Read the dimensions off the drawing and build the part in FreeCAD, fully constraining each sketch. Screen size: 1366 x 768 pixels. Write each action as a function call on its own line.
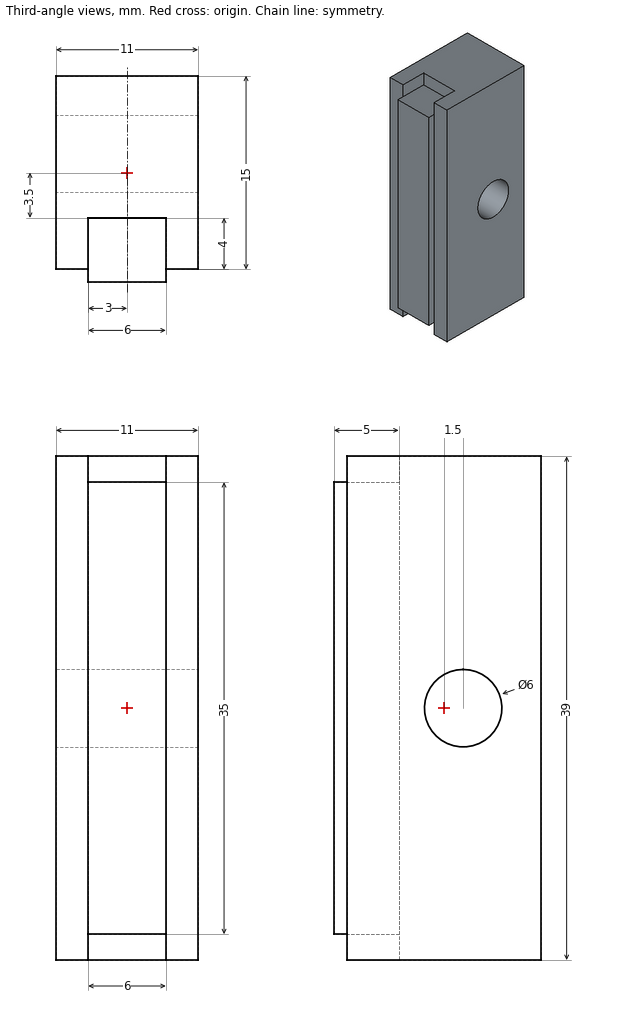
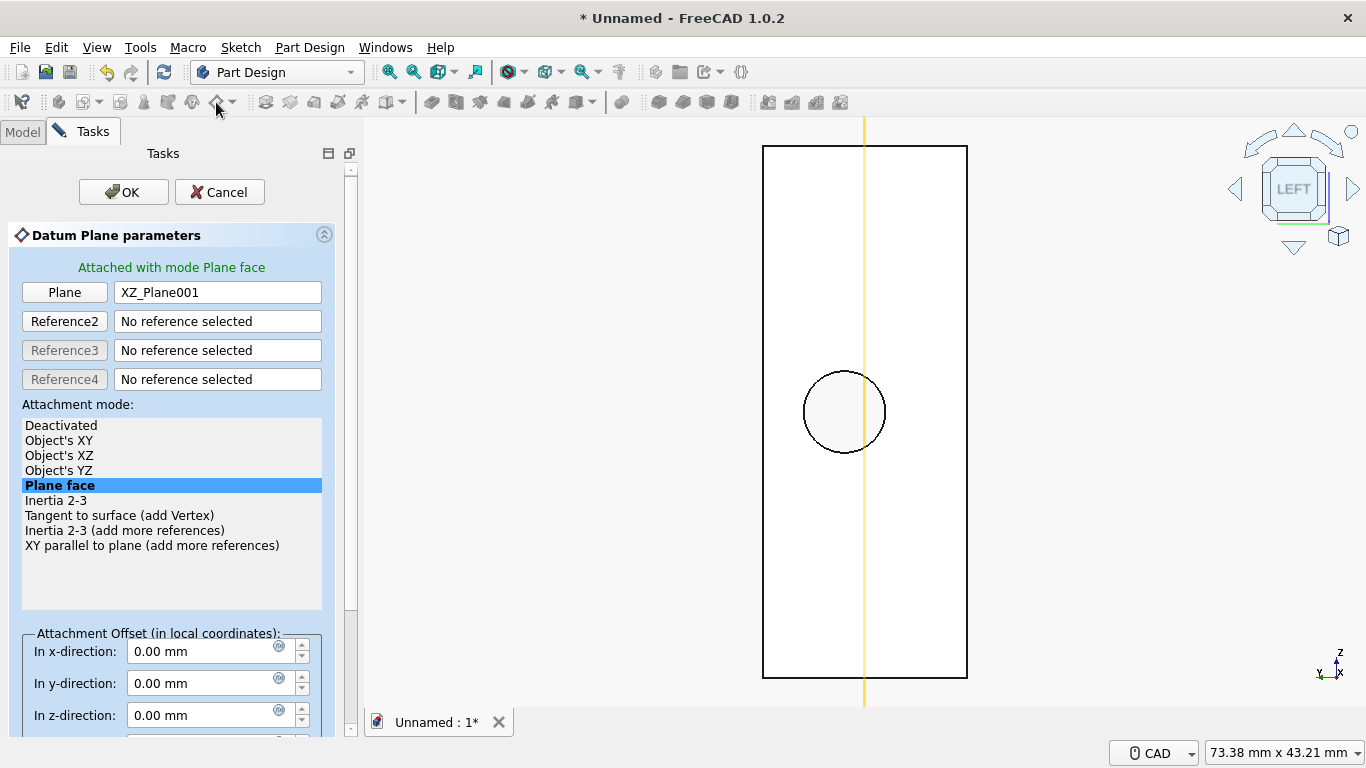
triple_click(210, 715)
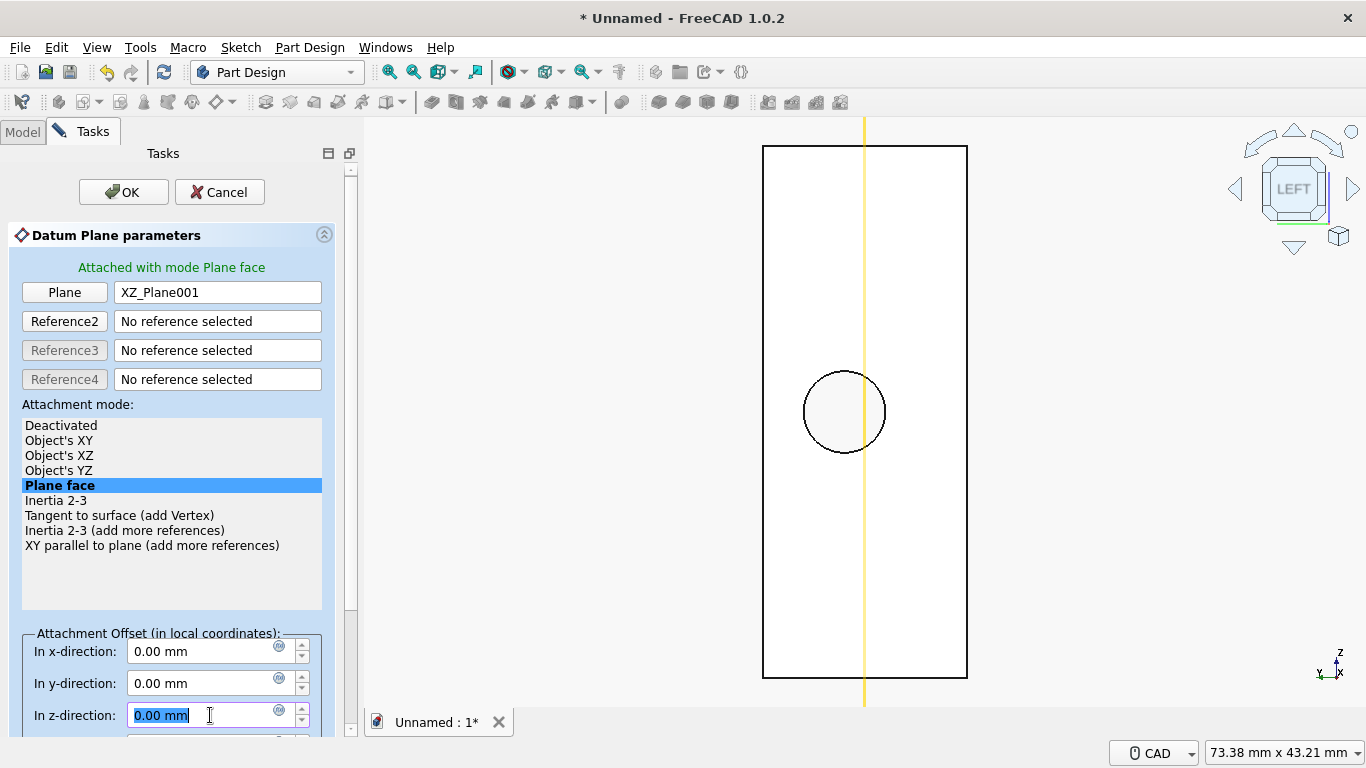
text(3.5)
key(Tab)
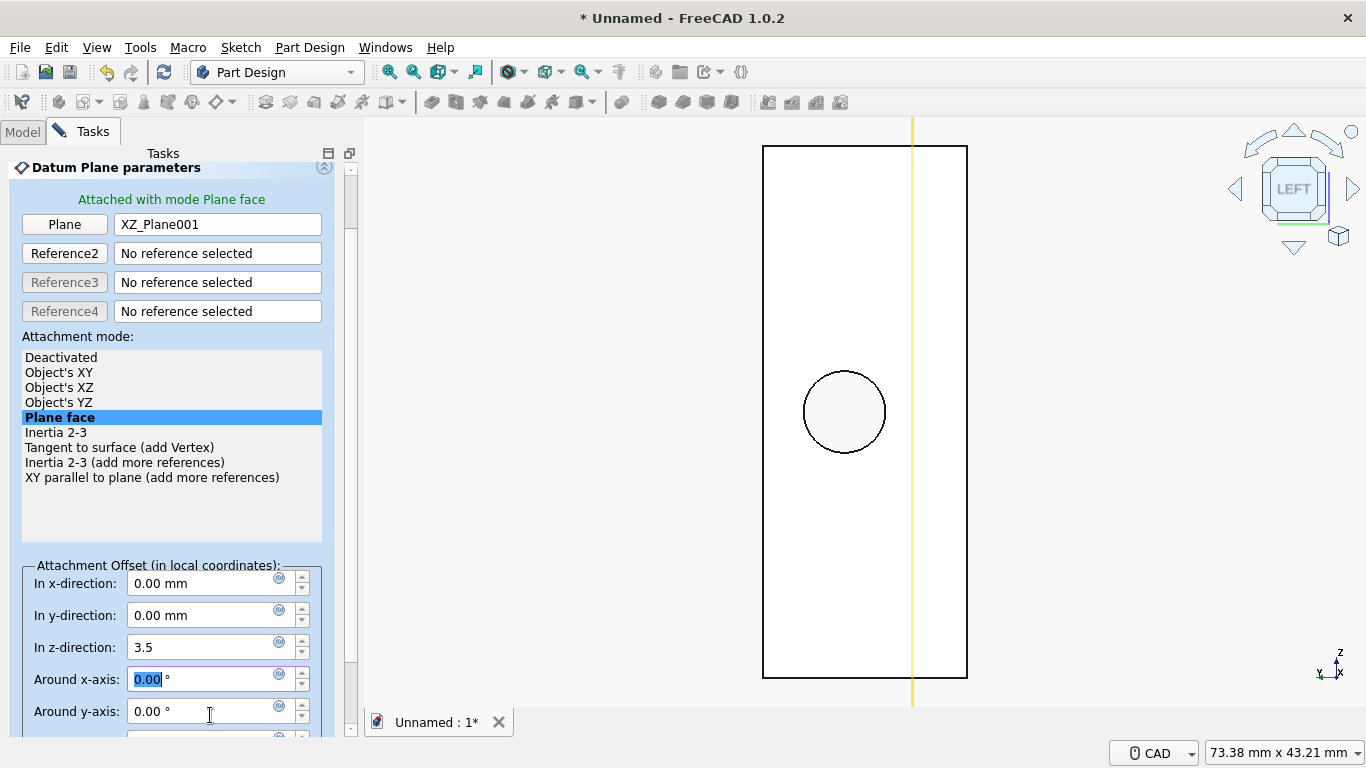
scroll(351, 450, up, 2)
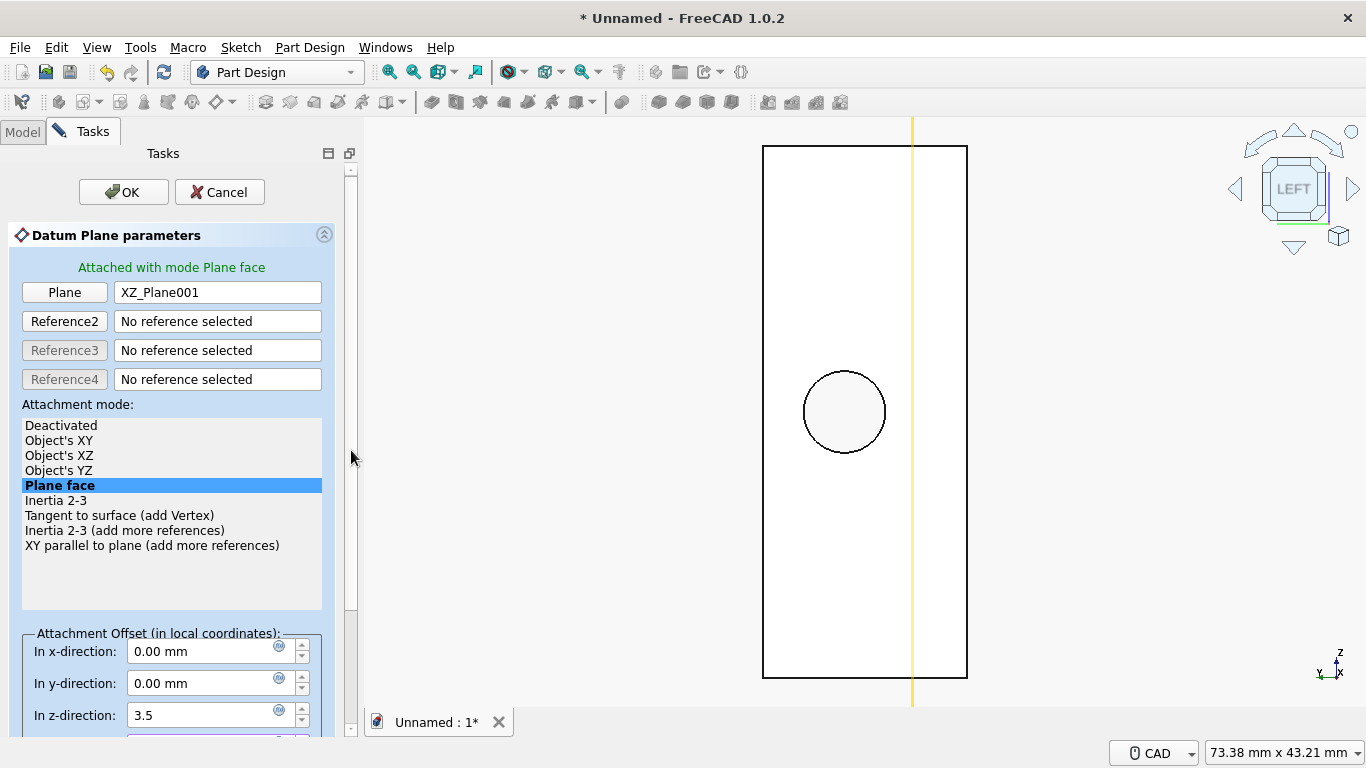
click(124, 192)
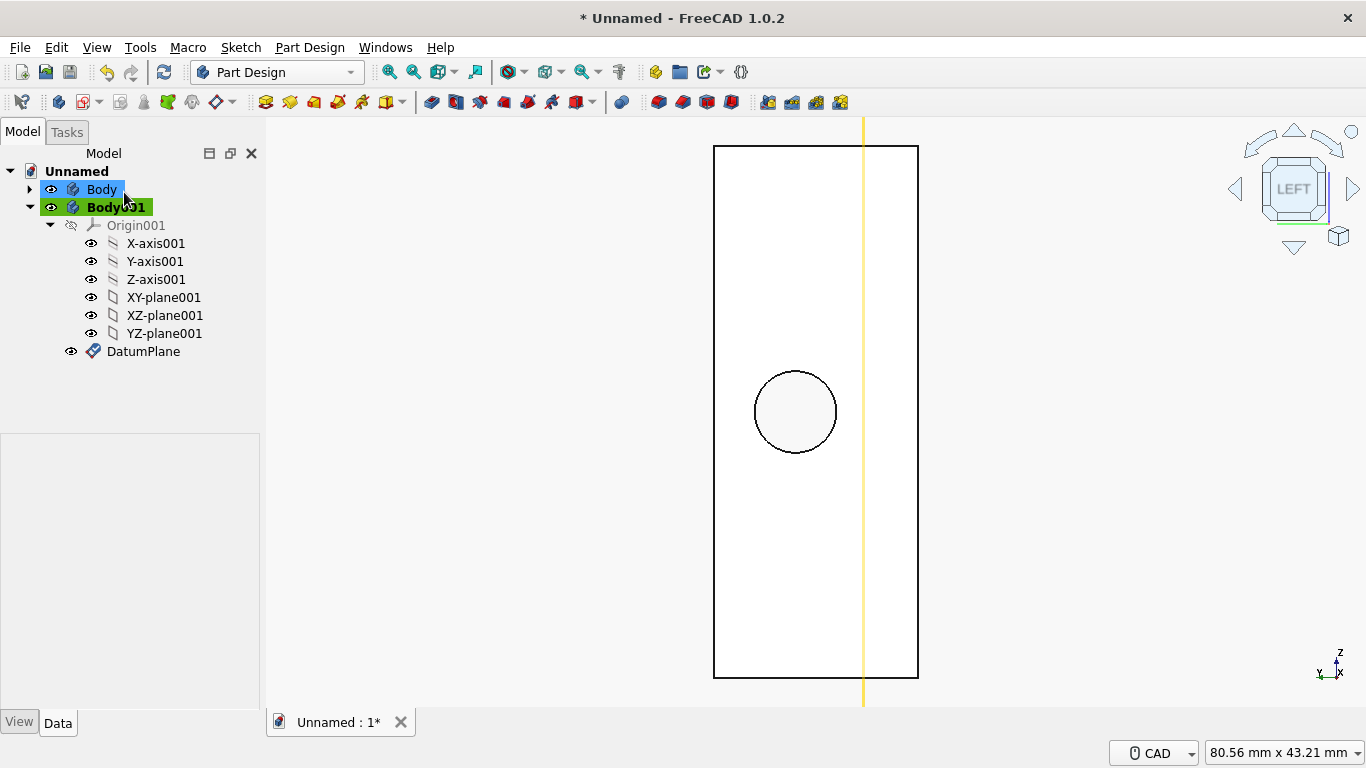
click(116, 351)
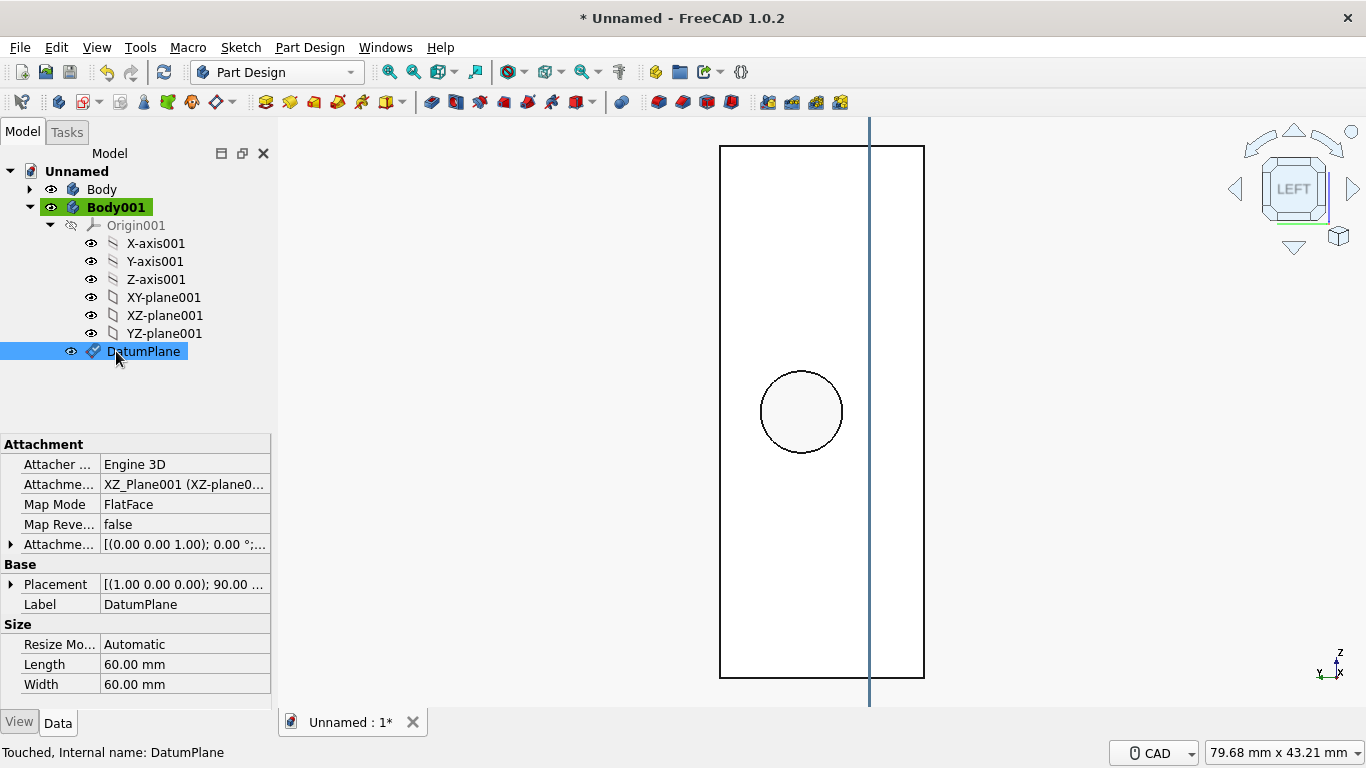
click(84, 102)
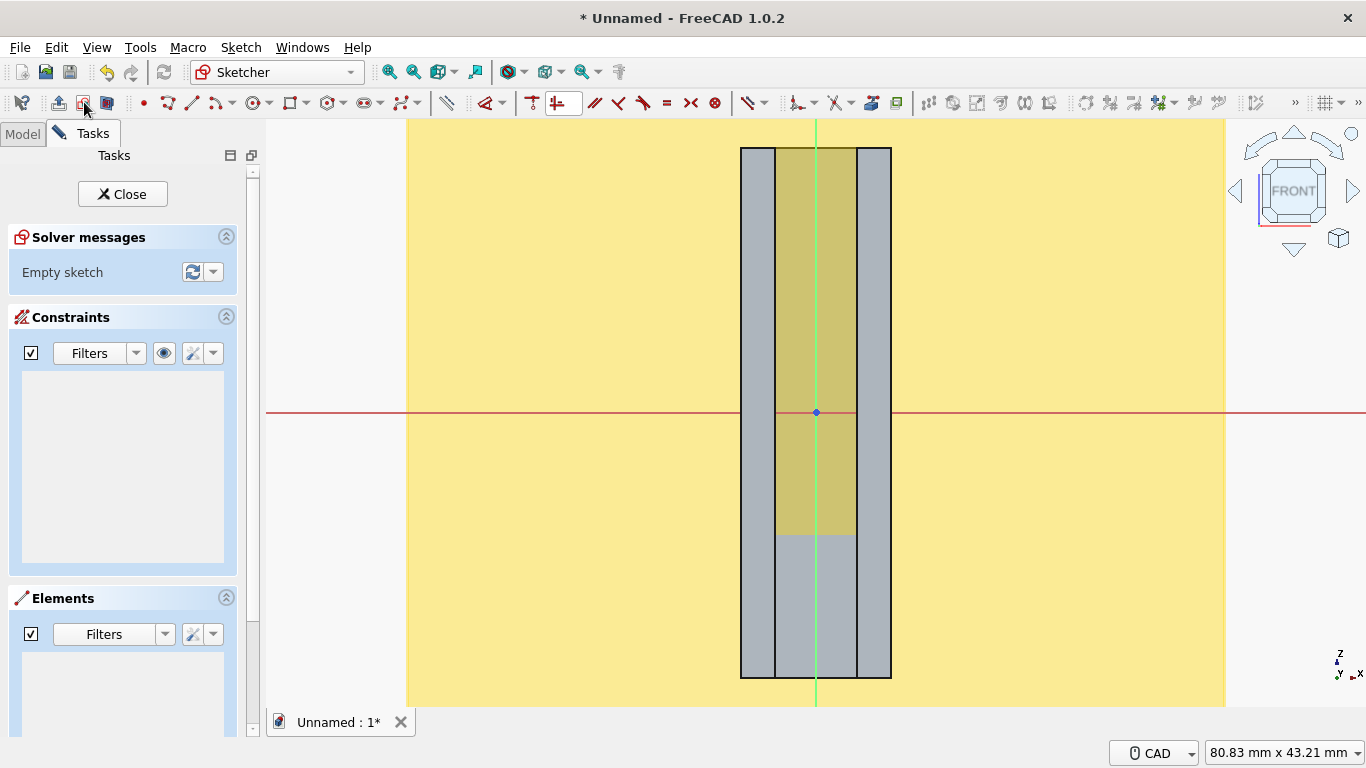
click(308, 104)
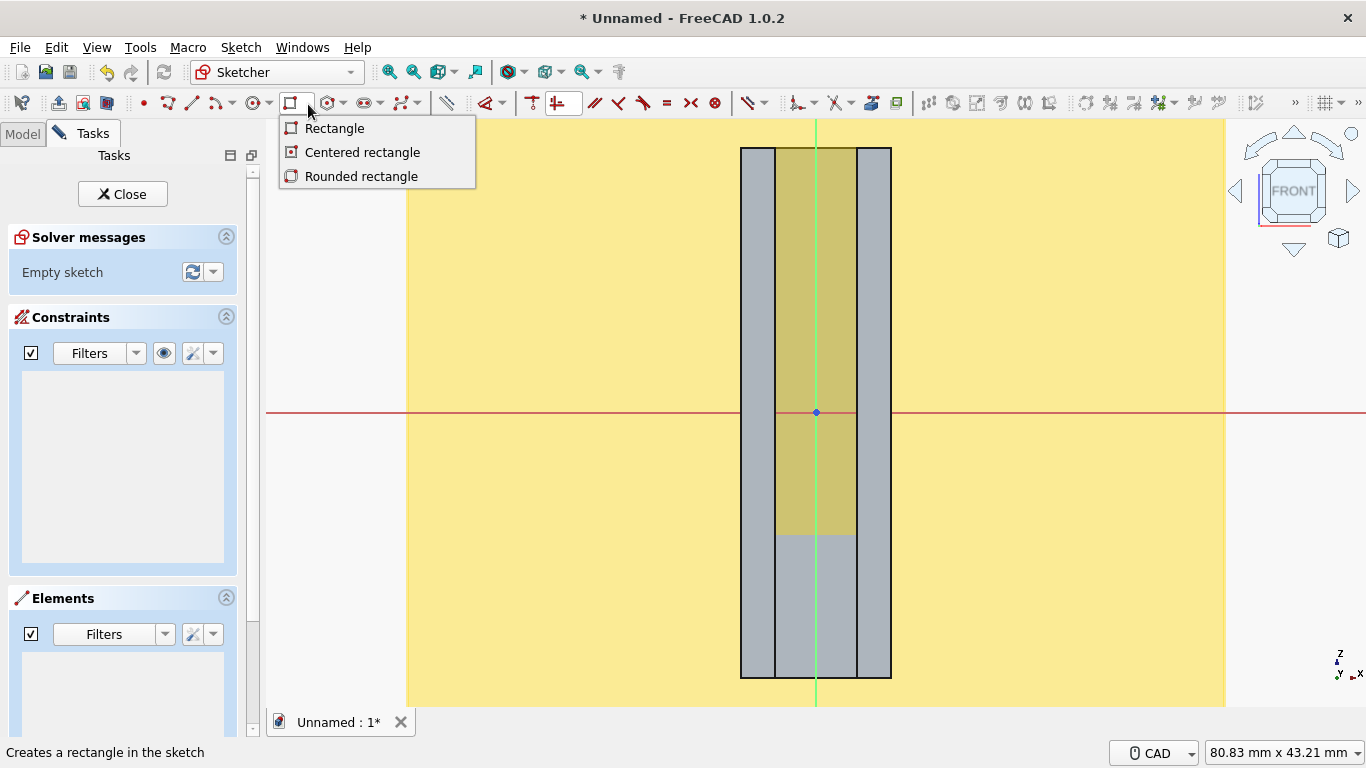
click(378, 152)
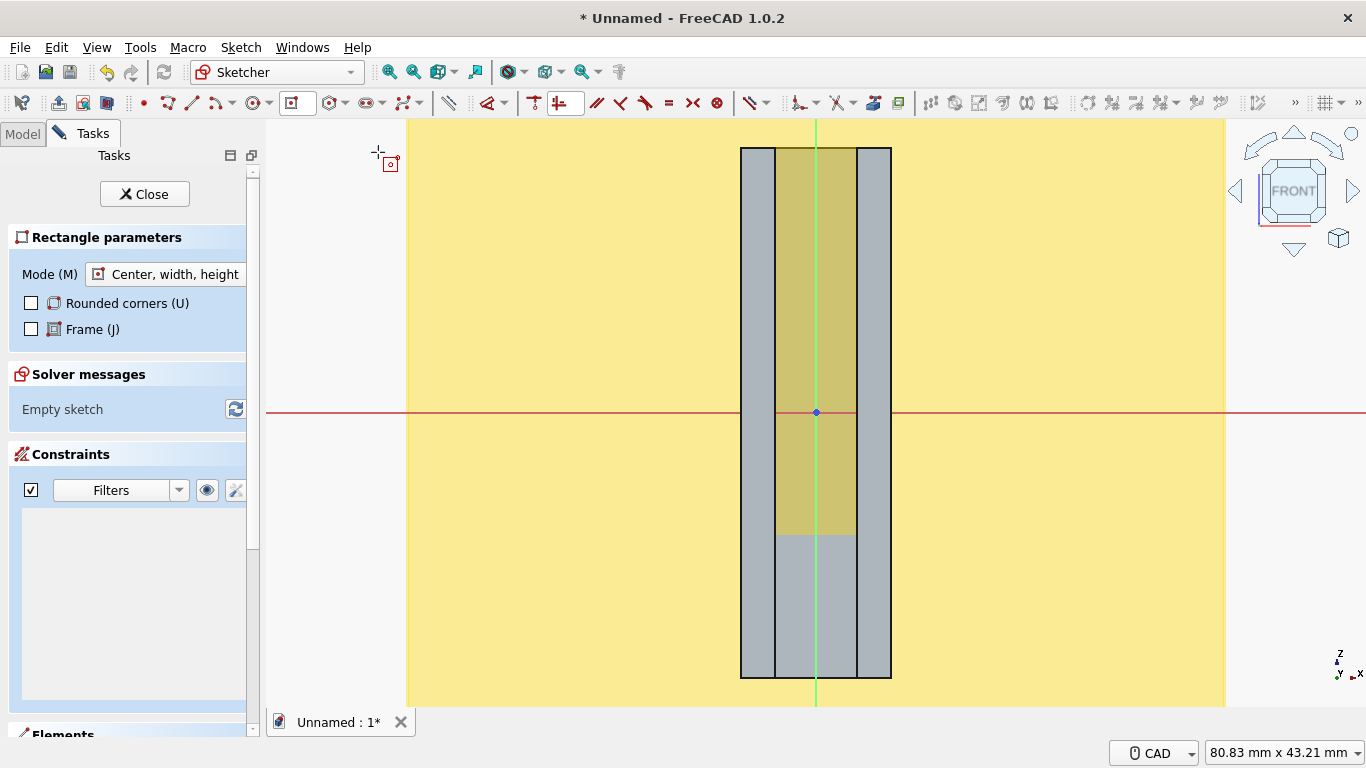
click(816, 413)
click(857, 175)
key(Escape)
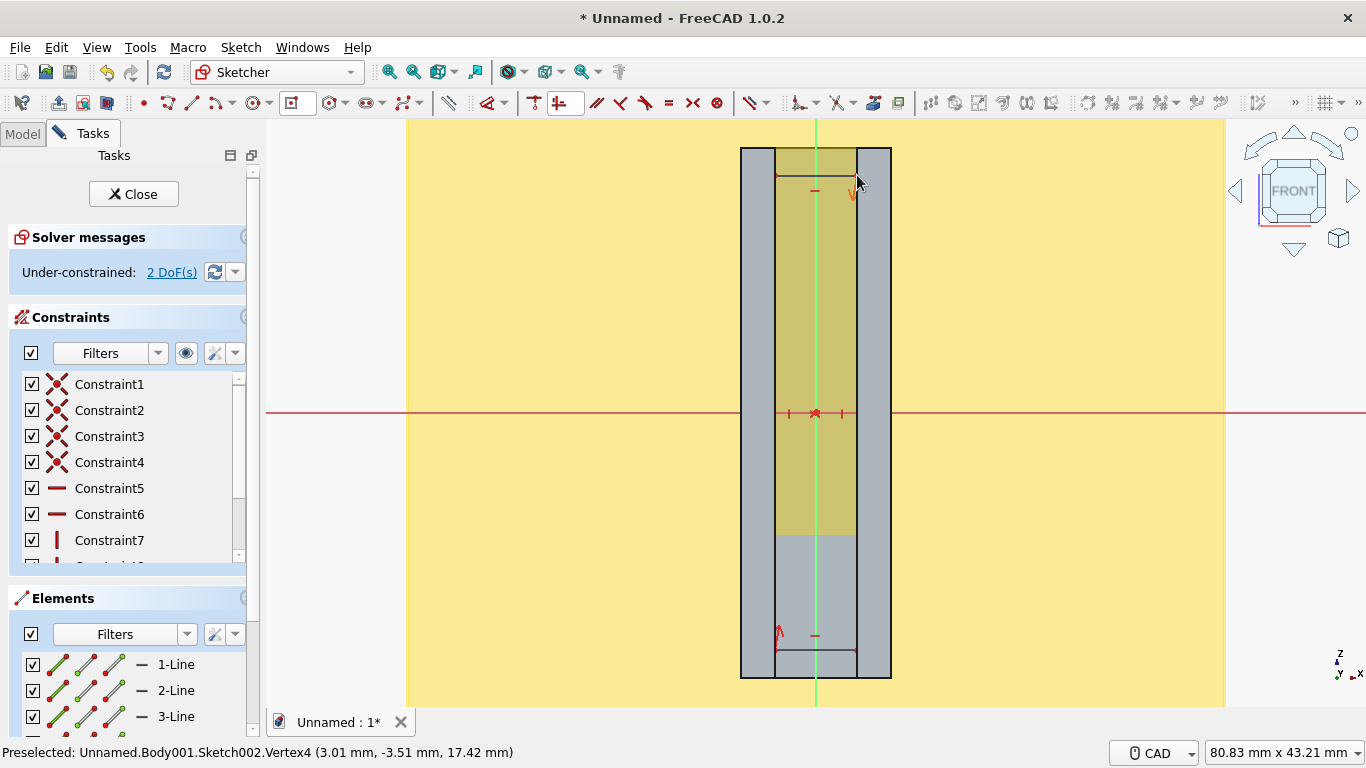
click(488, 104)